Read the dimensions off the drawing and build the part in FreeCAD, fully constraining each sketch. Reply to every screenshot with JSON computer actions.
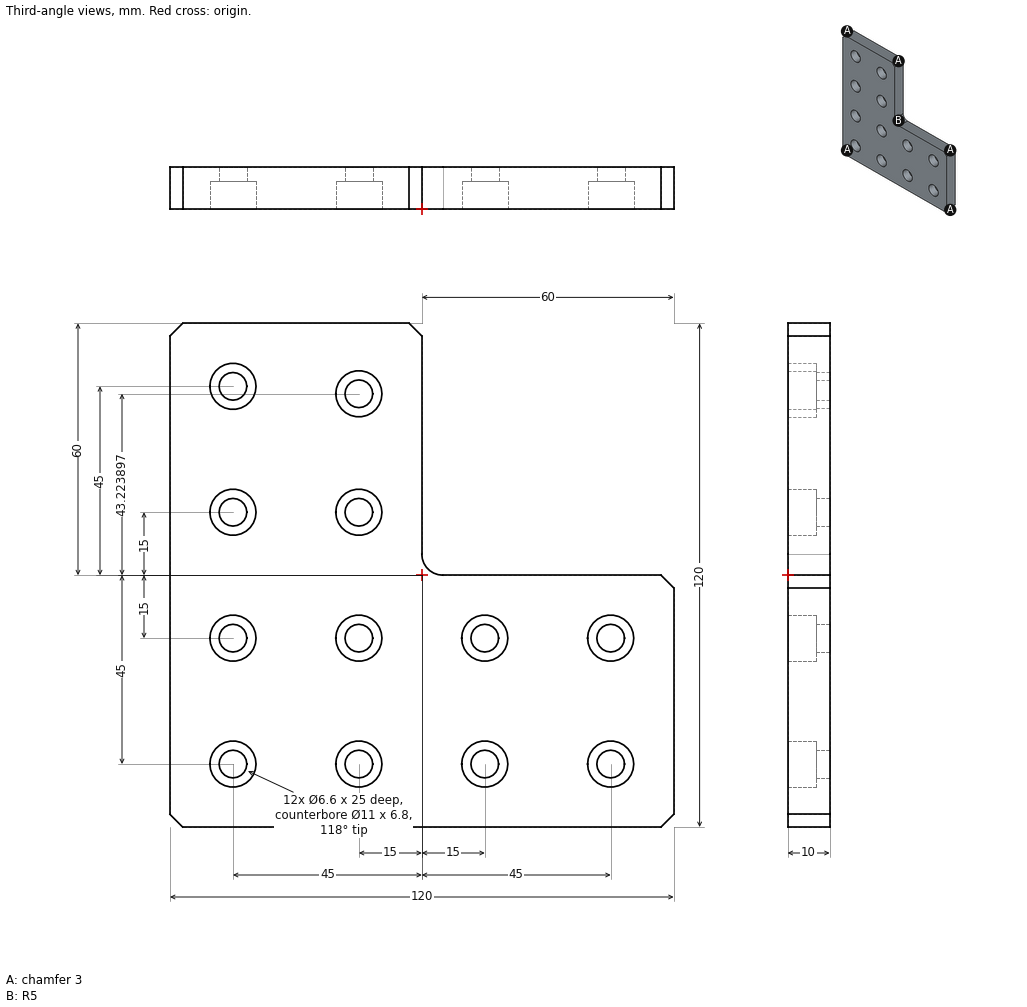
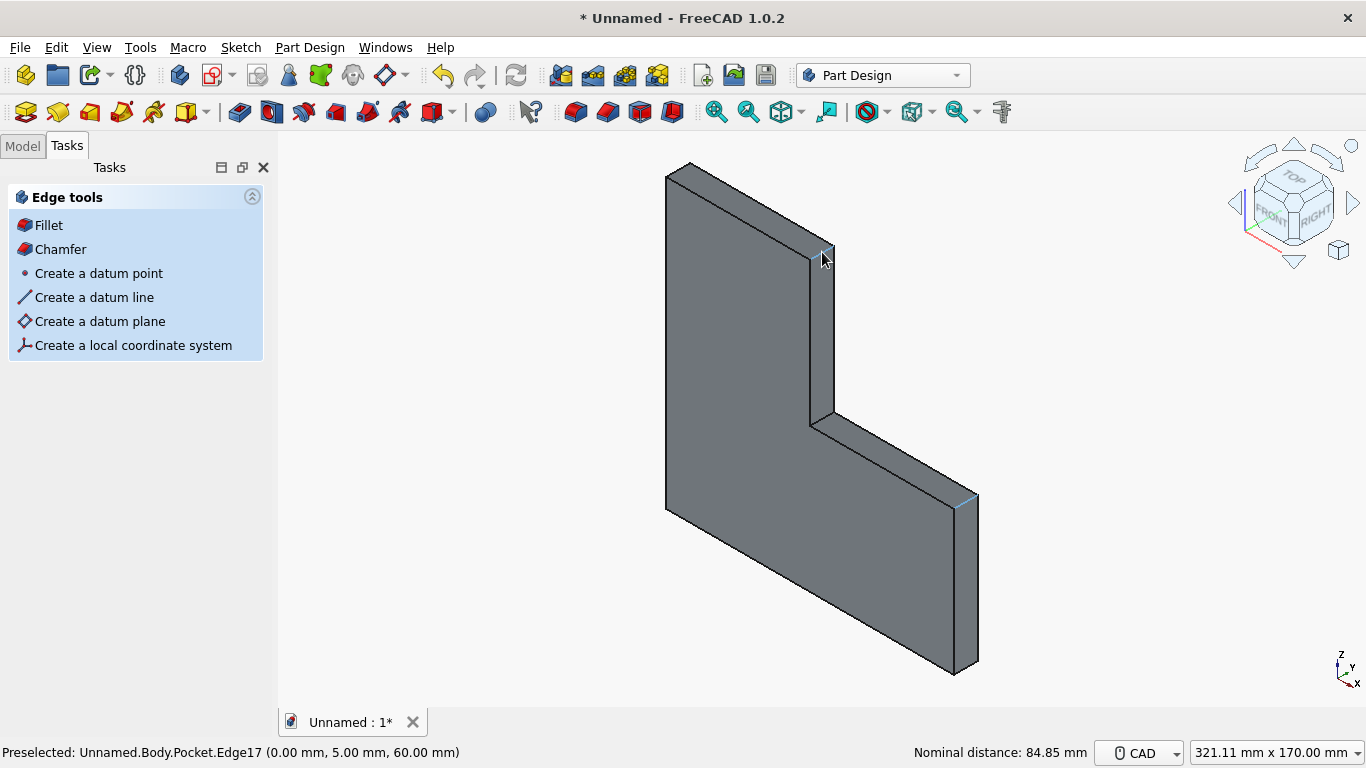
{"action": "key", "text": "2"}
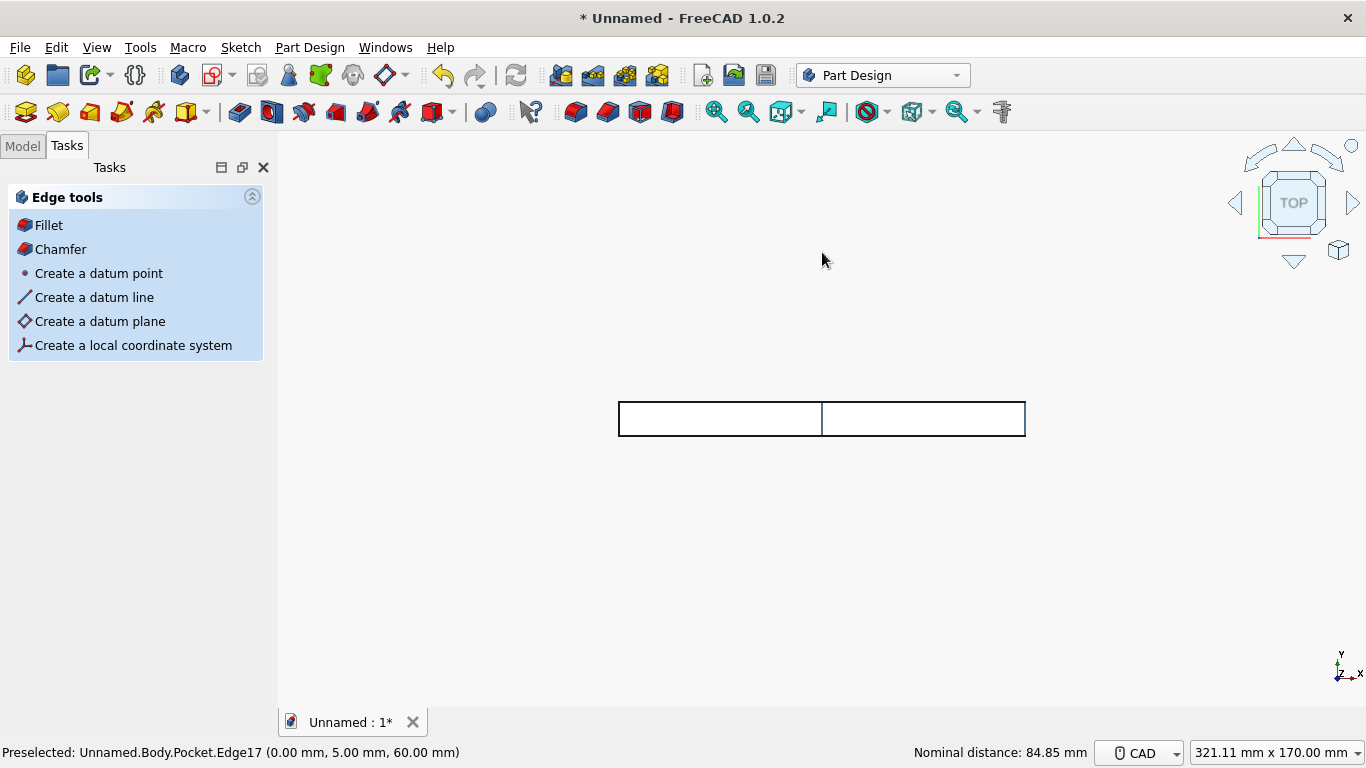
{"action": "left_click", "coordinate": [718, 112]}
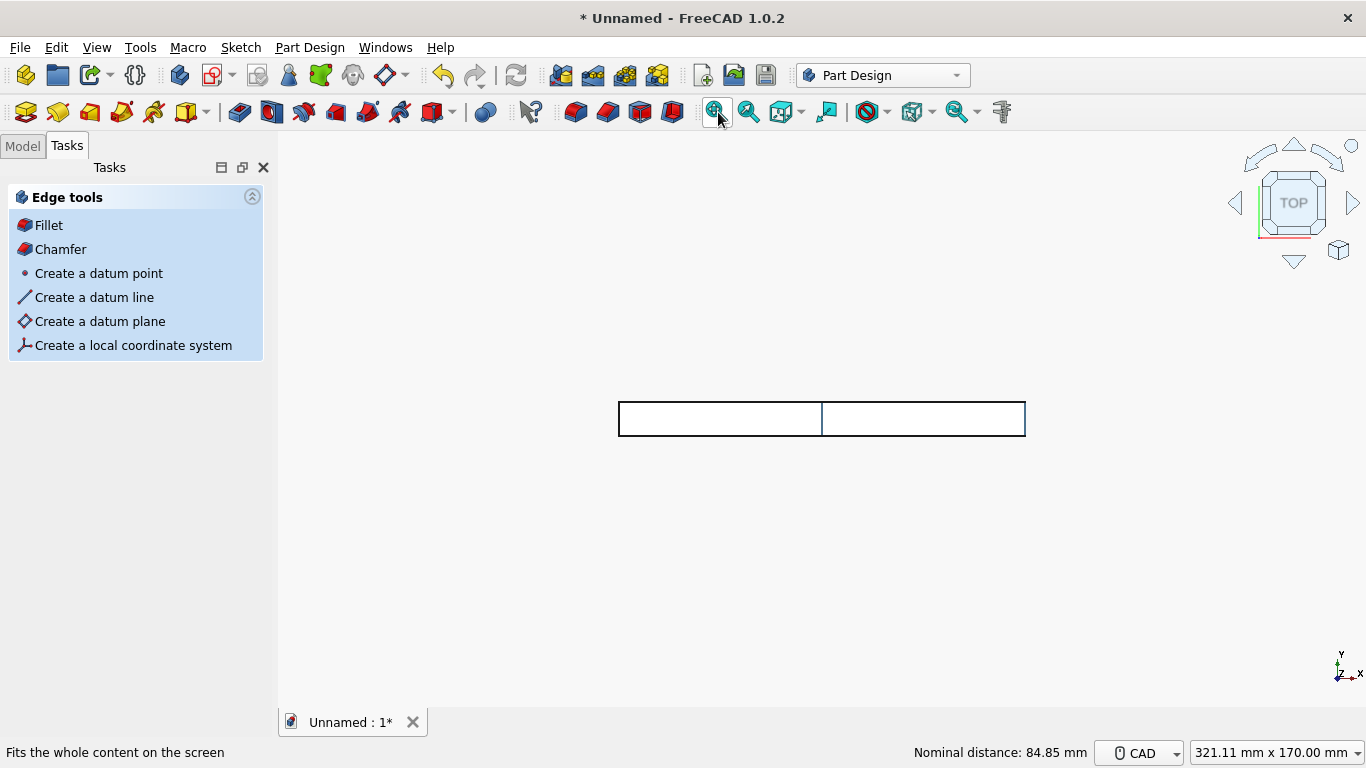
{"action": "left_click", "coordinate": [619, 418], "text": "ctrl"}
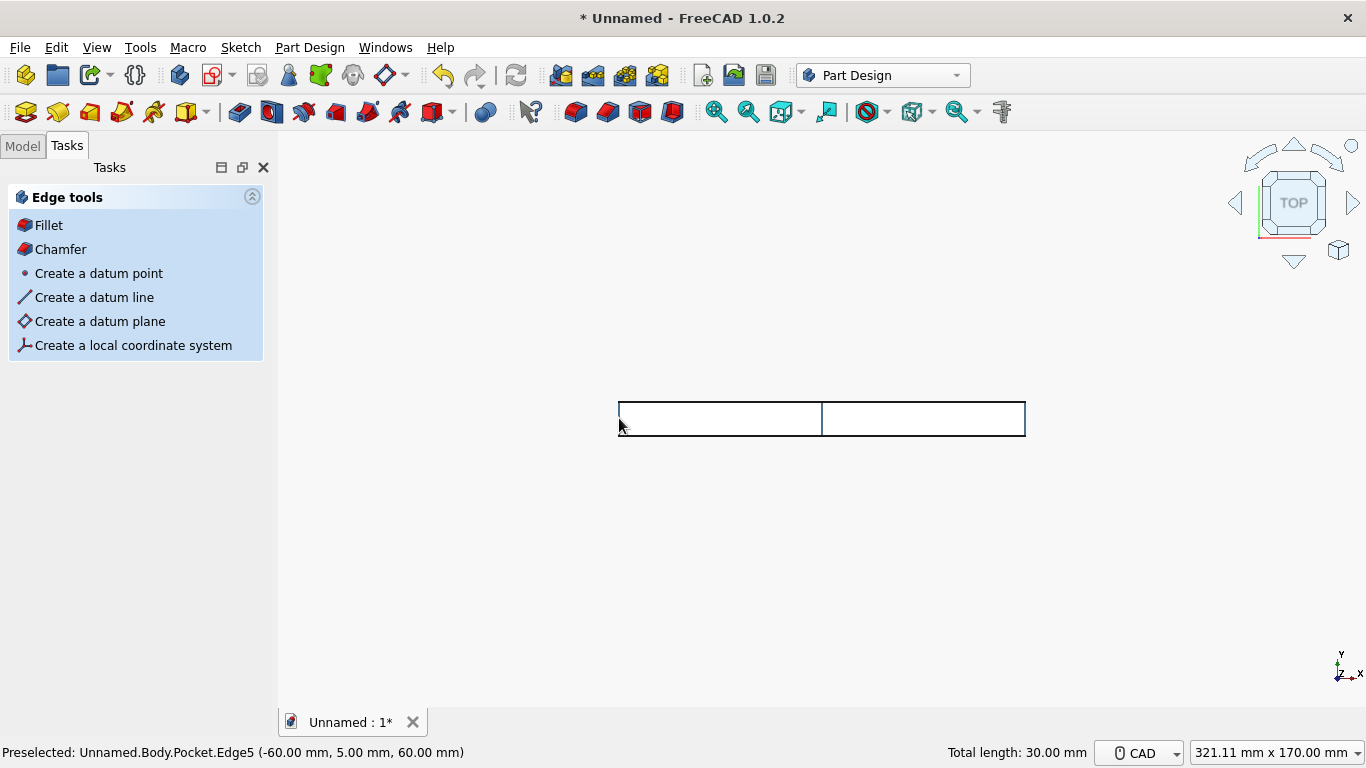
{"action": "key", "text": "1"}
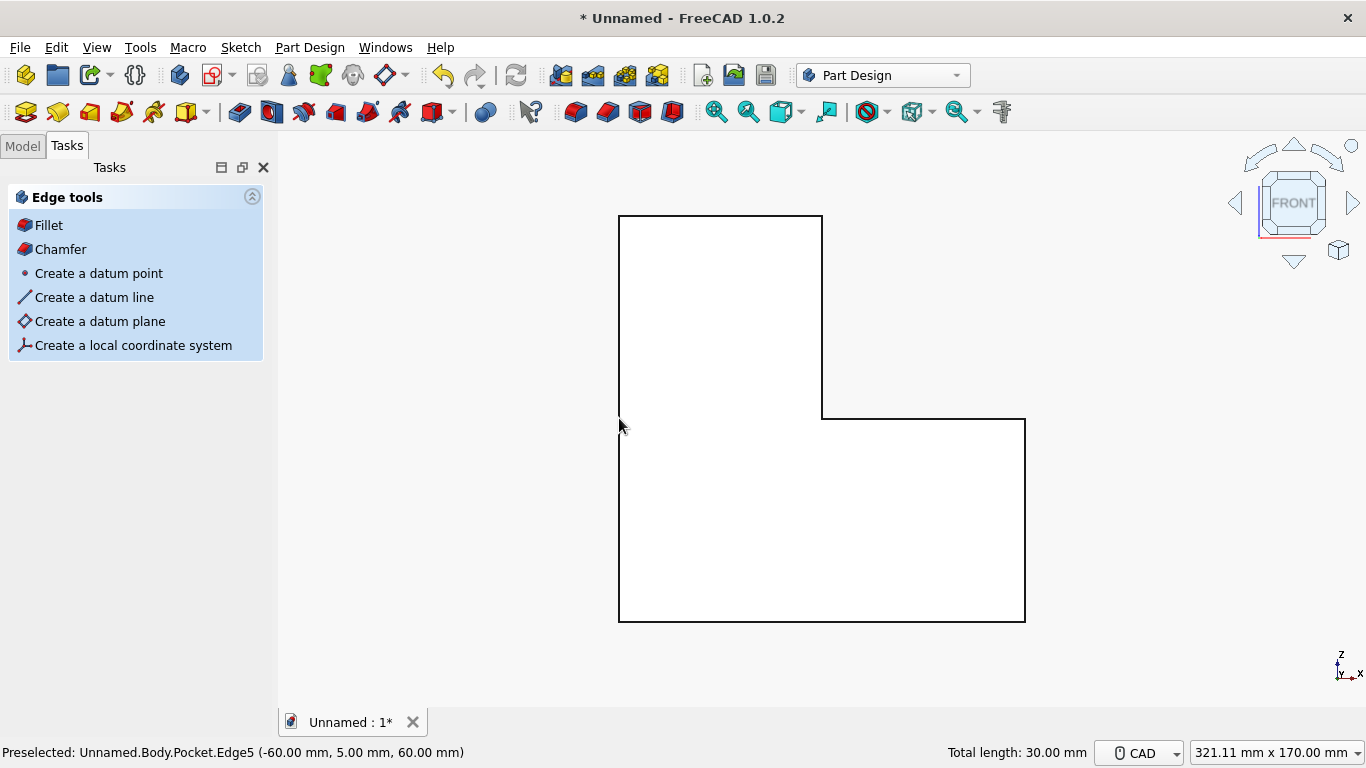
{"action": "key", "text": "3"}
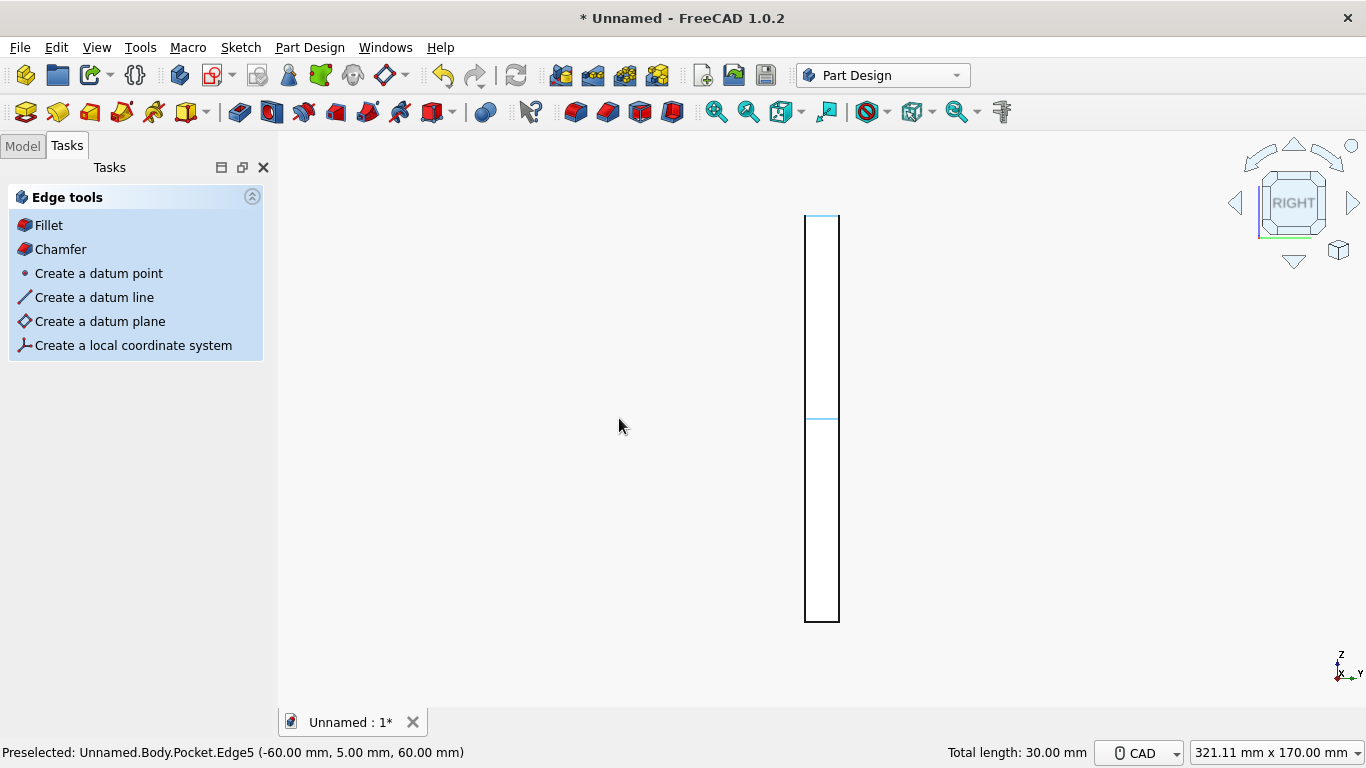
{"action": "left_click", "coordinate": [822, 621], "text": "ctrl"}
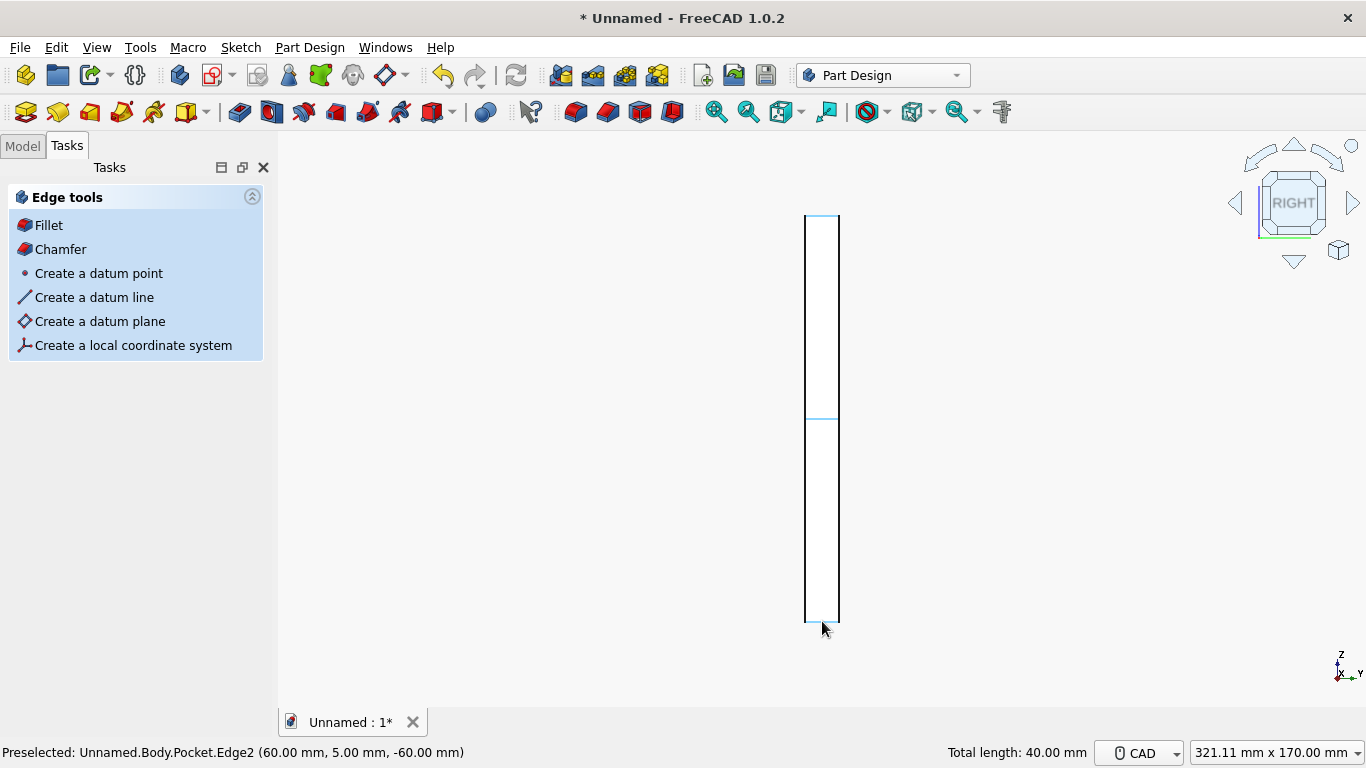
{"action": "key", "text": "5"}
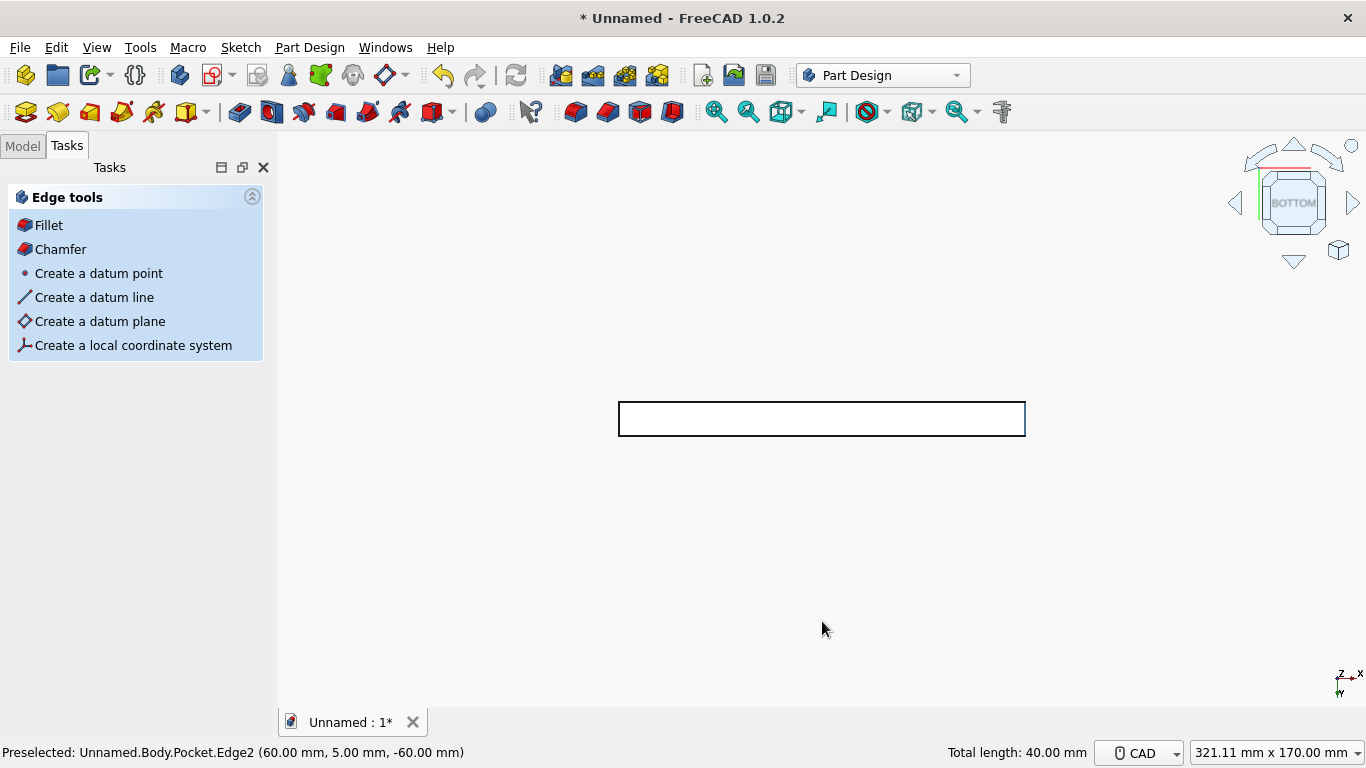
{"action": "left_click", "coordinate": [718, 112]}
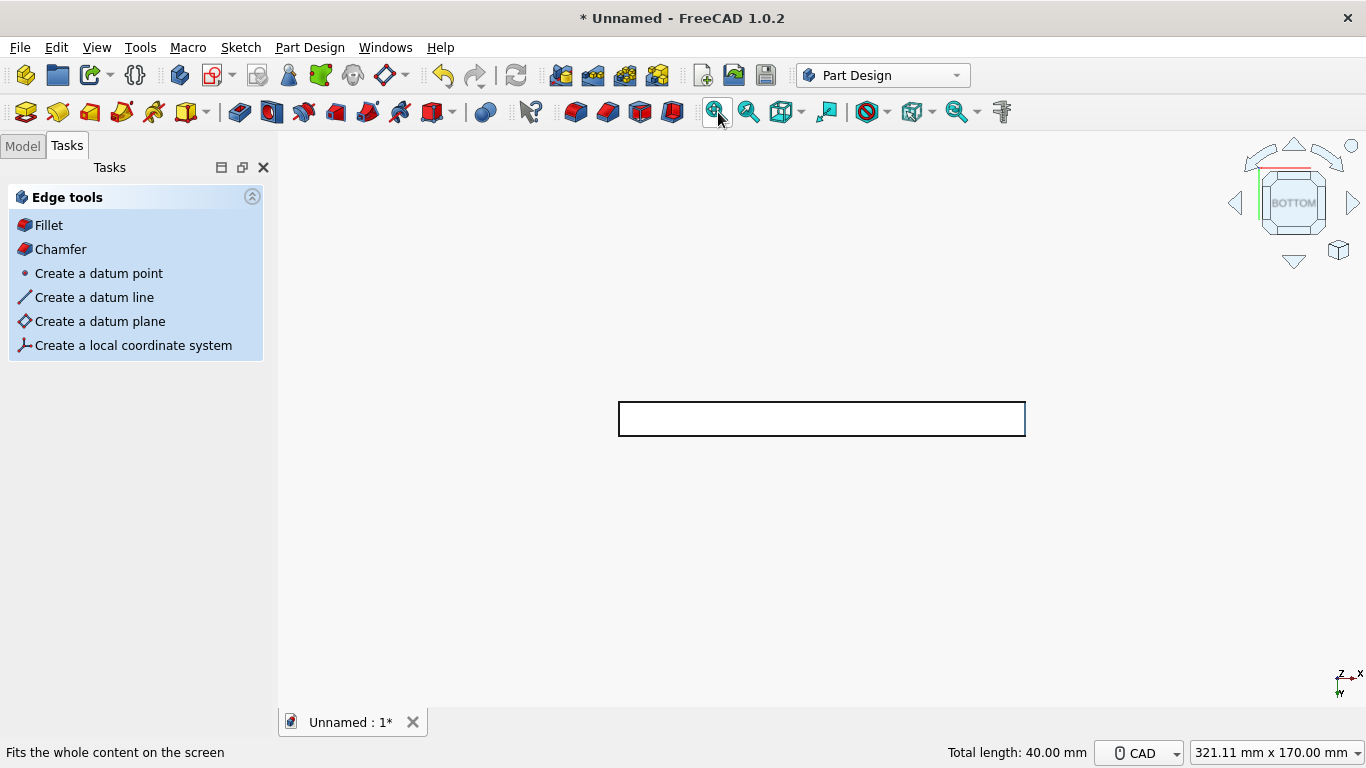
{"action": "left_click", "coordinate": [619, 418], "text": "ctrl"}